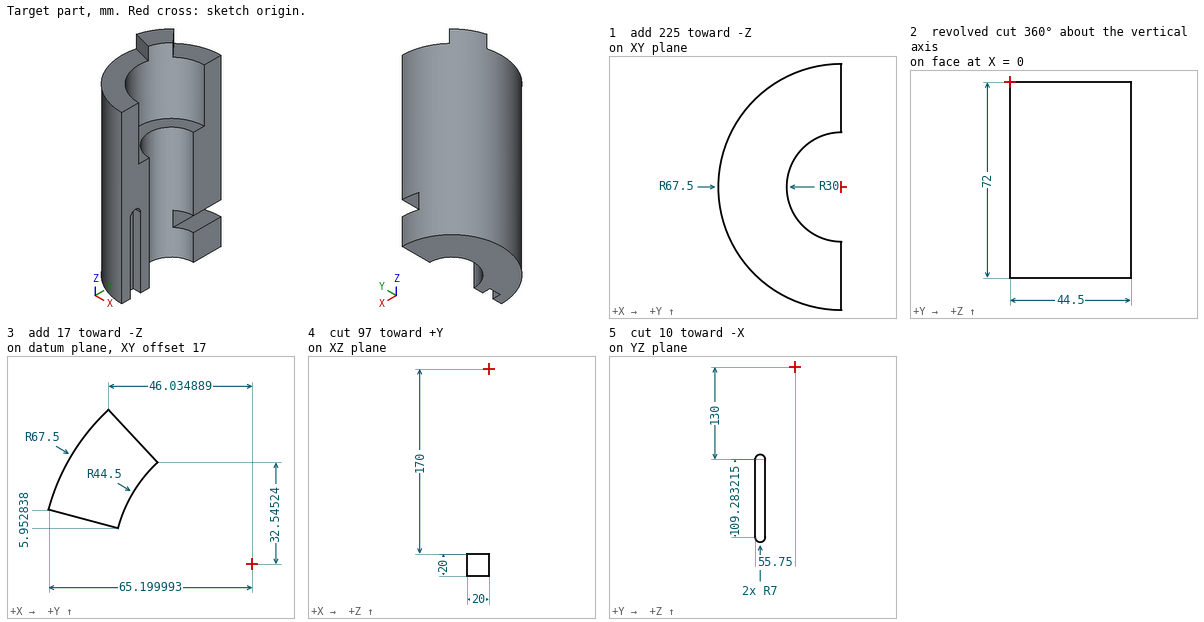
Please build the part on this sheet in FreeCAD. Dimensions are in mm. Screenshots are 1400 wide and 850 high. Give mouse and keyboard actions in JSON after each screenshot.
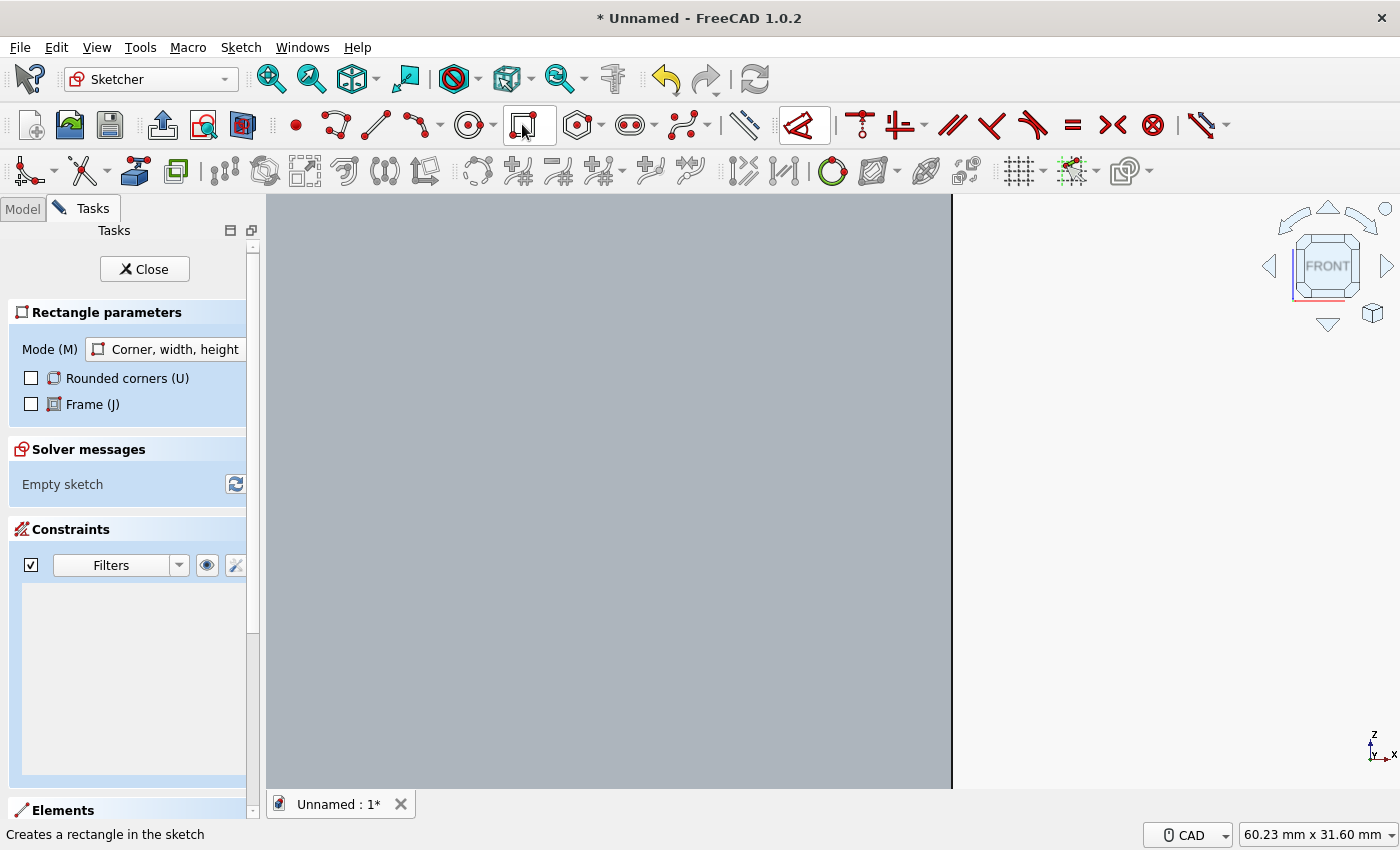
{"action": "left_click", "coordinate": [576, 300]}
{"action": "left_click", "coordinate": [952, 677]}
{"action": "key", "text": "Escape"}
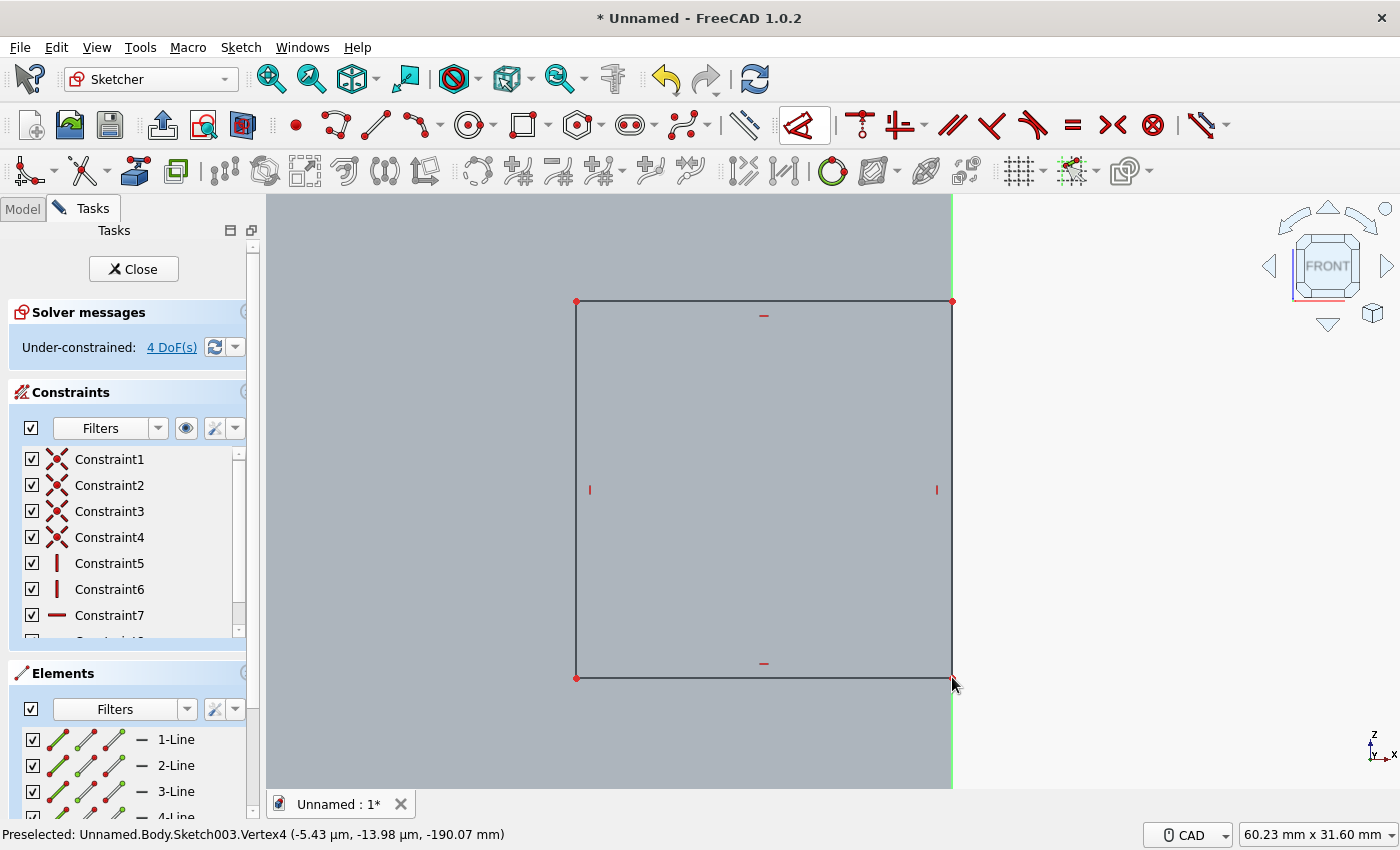
{"action": "left_click", "coordinate": [952, 678]}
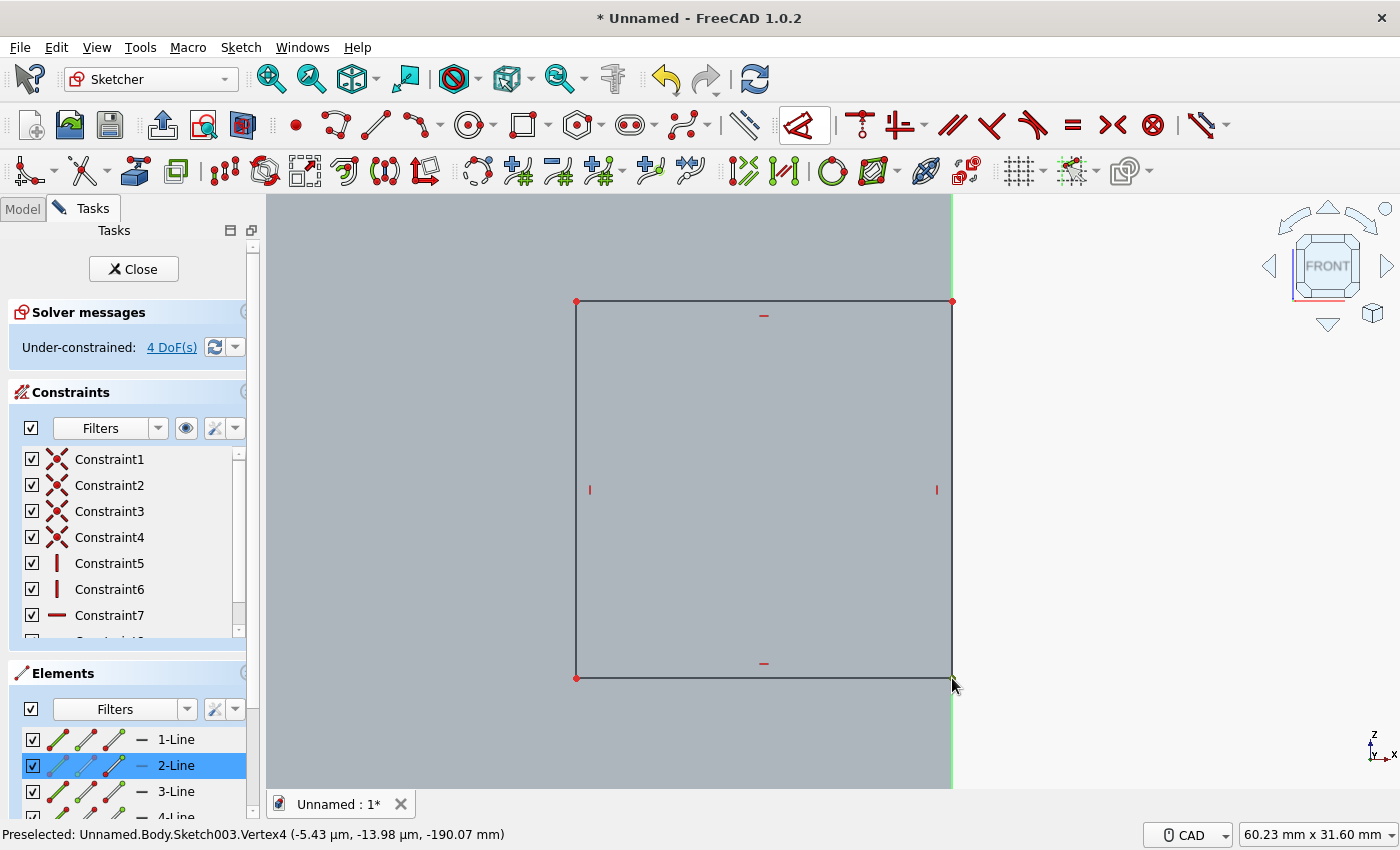
{"action": "left_click", "coordinate": [952, 722]}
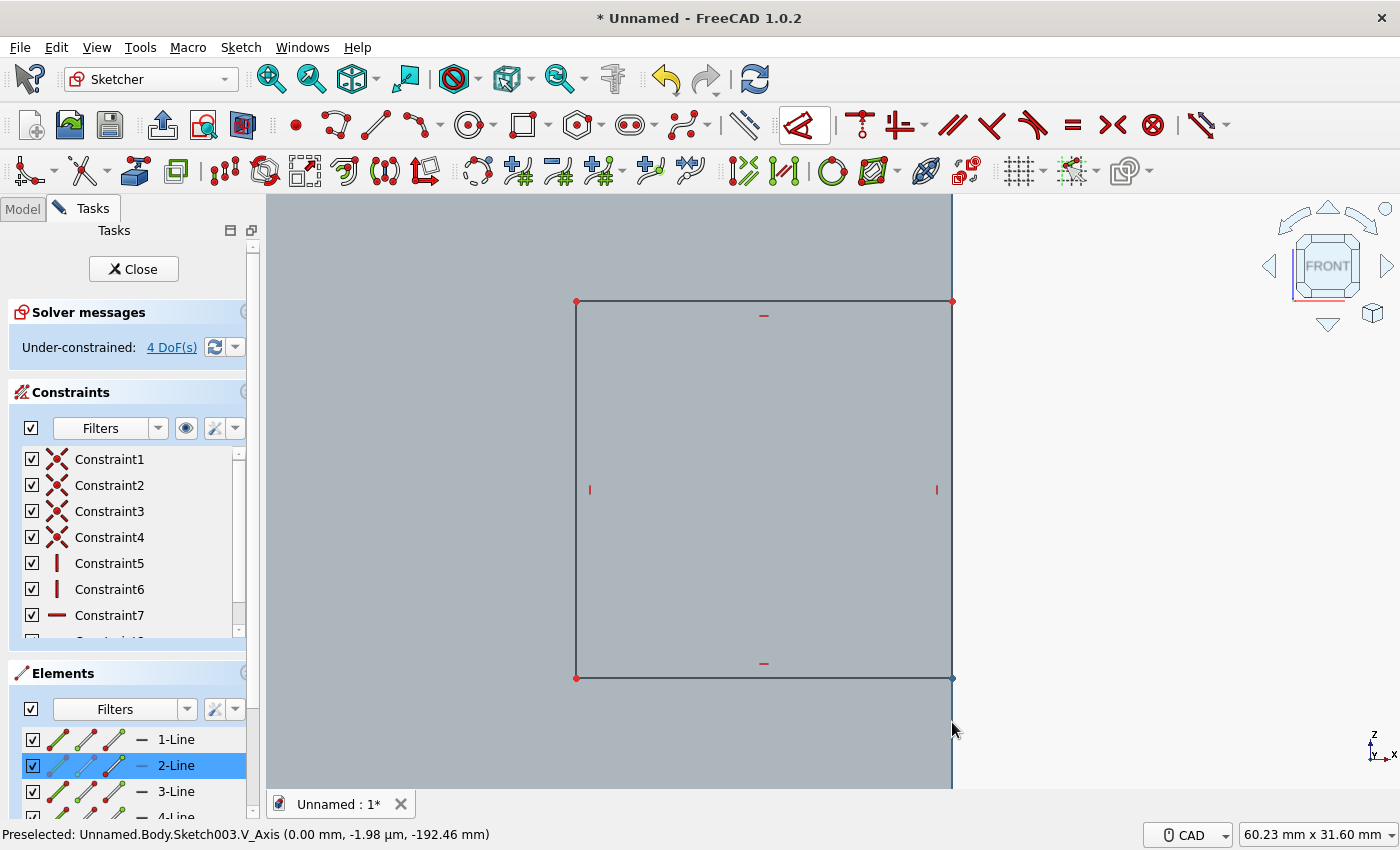
{"action": "left_click", "coordinate": [860, 126]}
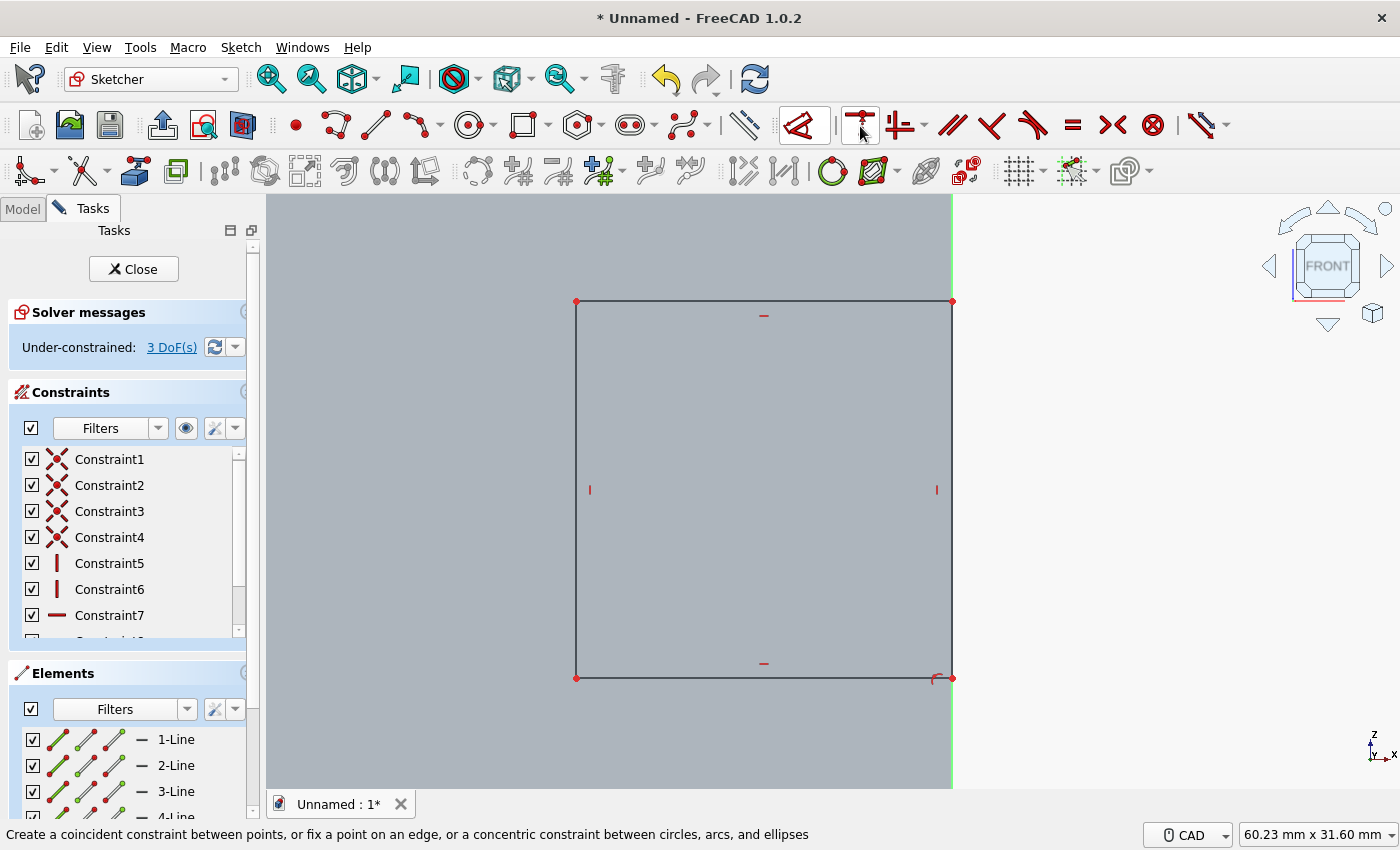
{"action": "left_click", "coordinate": [576, 414]}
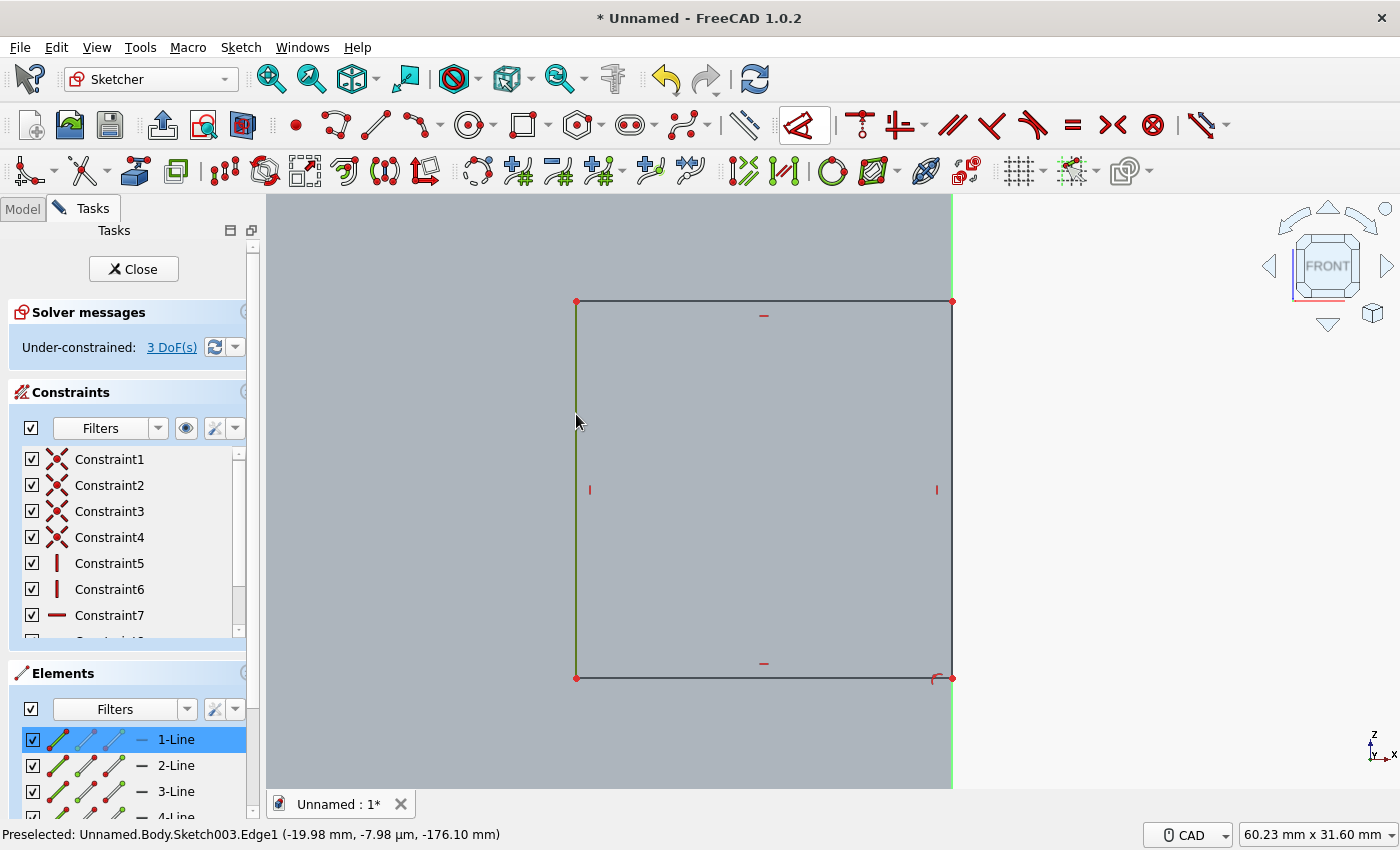
{"action": "left_click", "coordinate": [824, 126]}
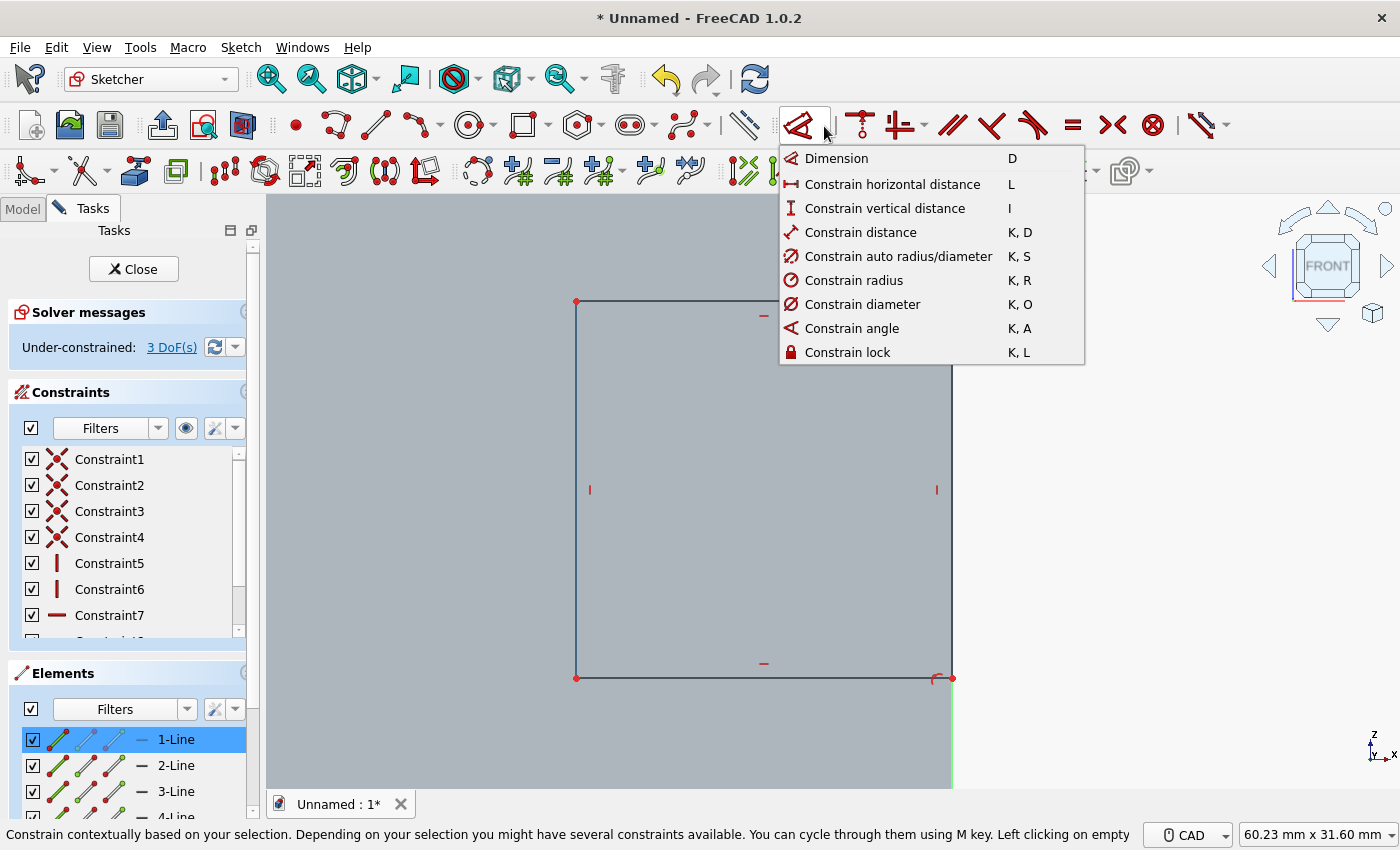
{"action": "left_click", "coordinate": [932, 208]}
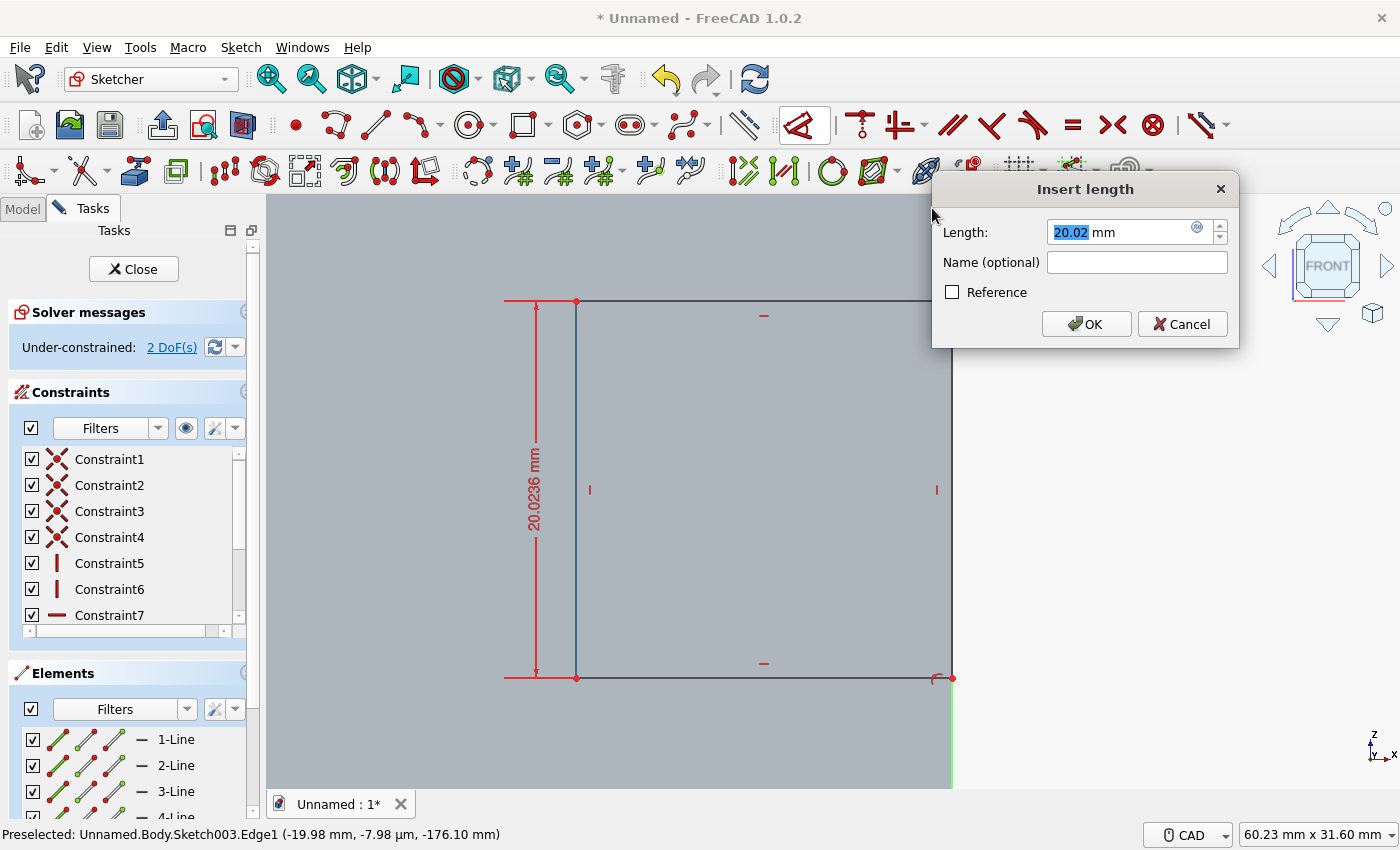
{"action": "type", "text": "20"}
{"action": "key", "text": "Return"}